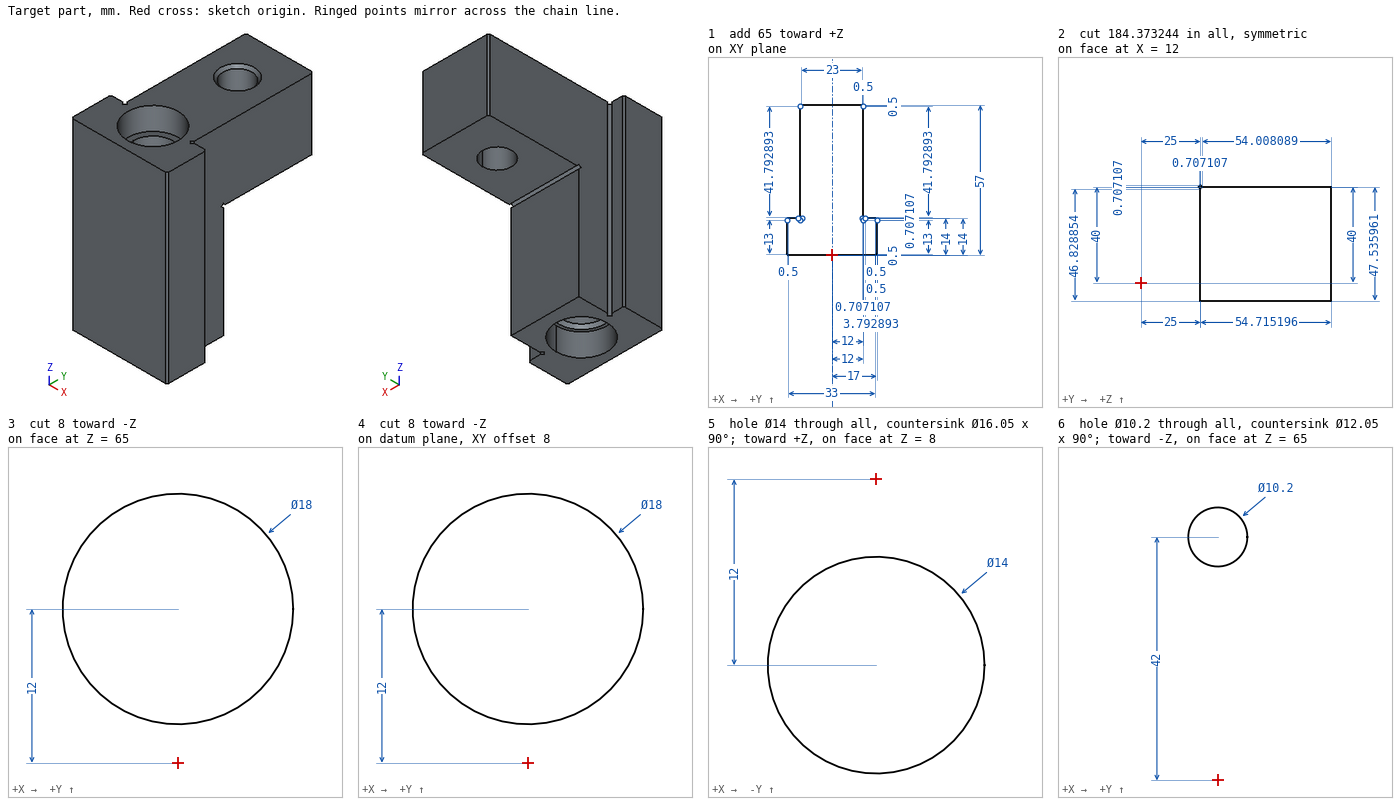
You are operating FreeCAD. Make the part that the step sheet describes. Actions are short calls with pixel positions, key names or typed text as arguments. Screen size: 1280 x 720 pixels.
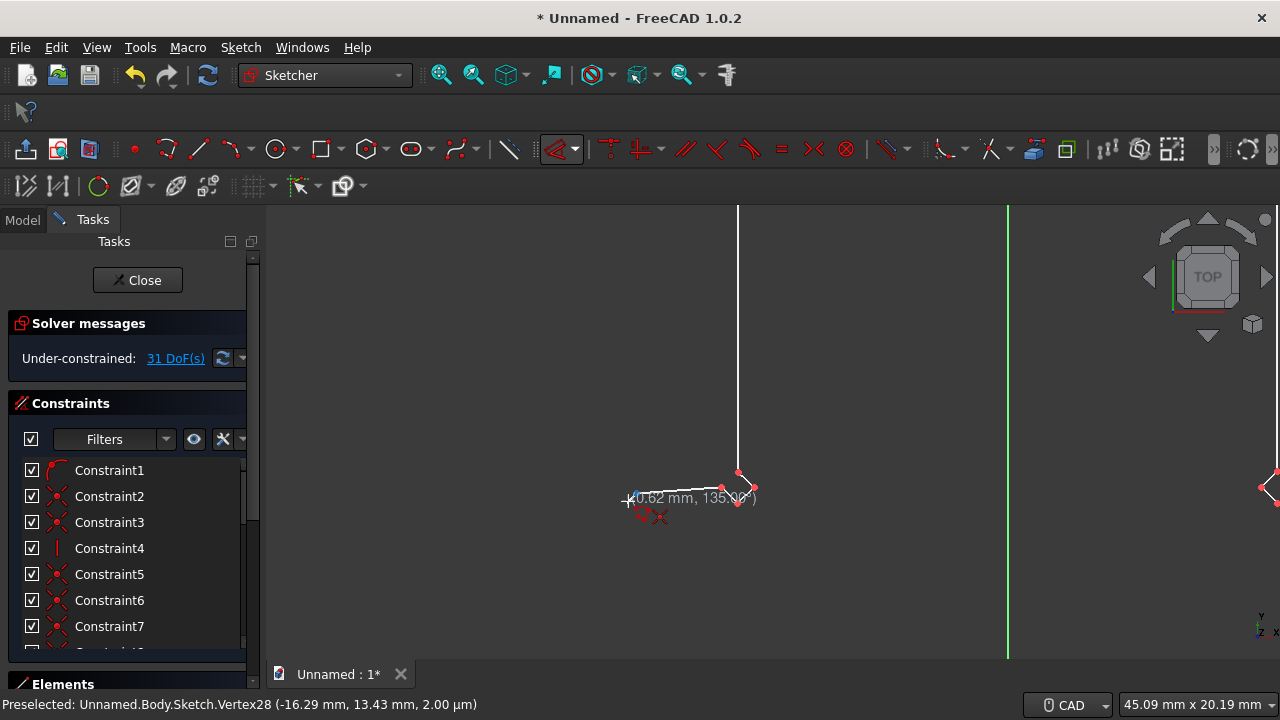
click(625, 497)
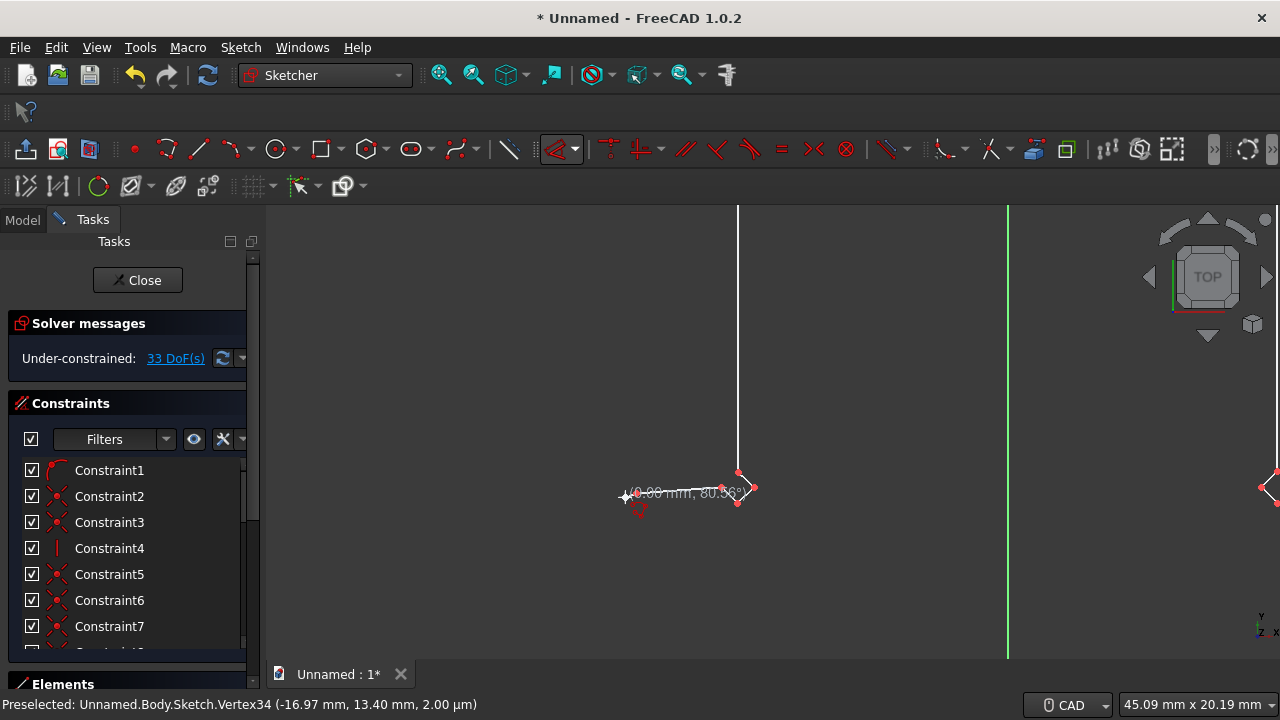
scroll(628, 501, down, 8)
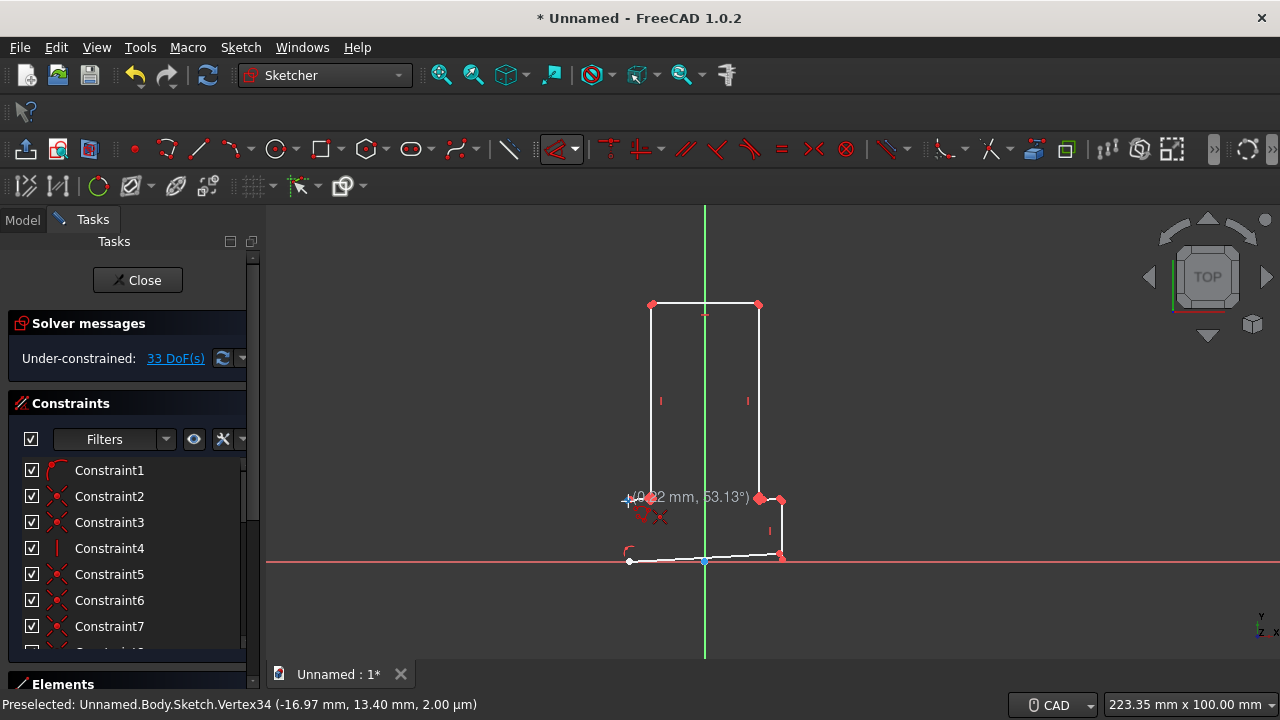
scroll(628, 560, up, 10)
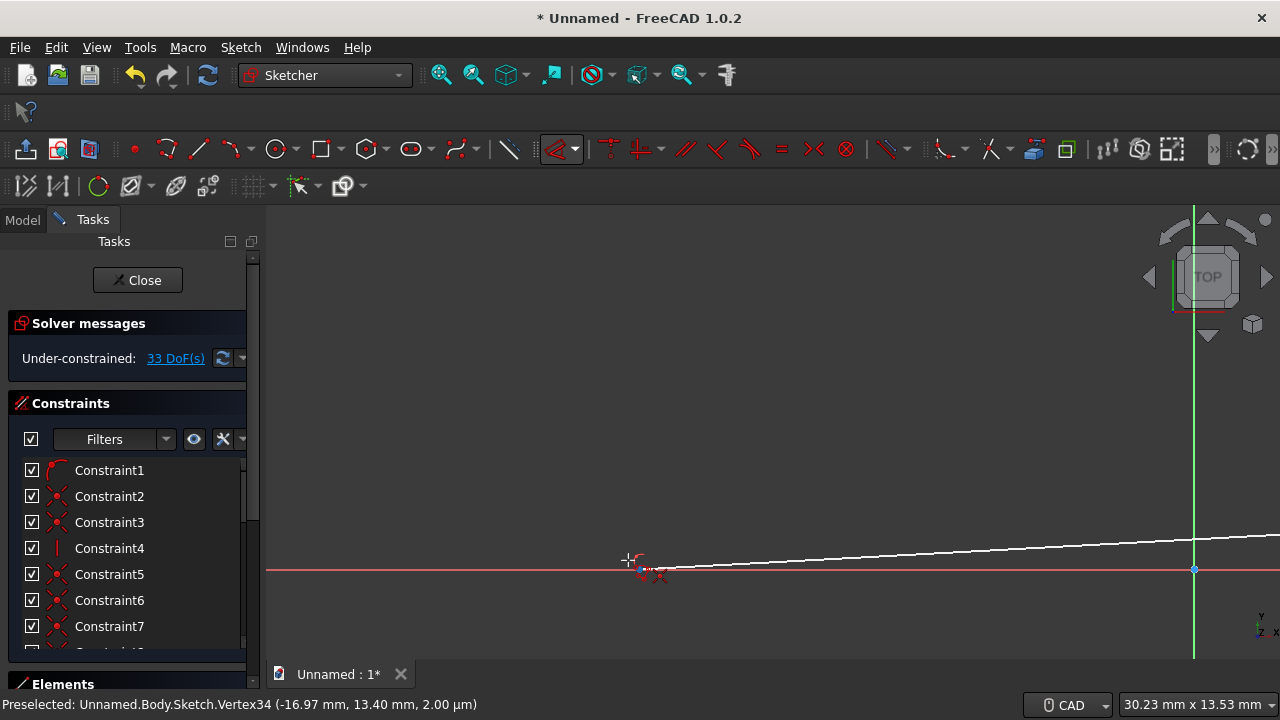
click(623, 553)
click(640, 570)
key(Escape)
key(Escape)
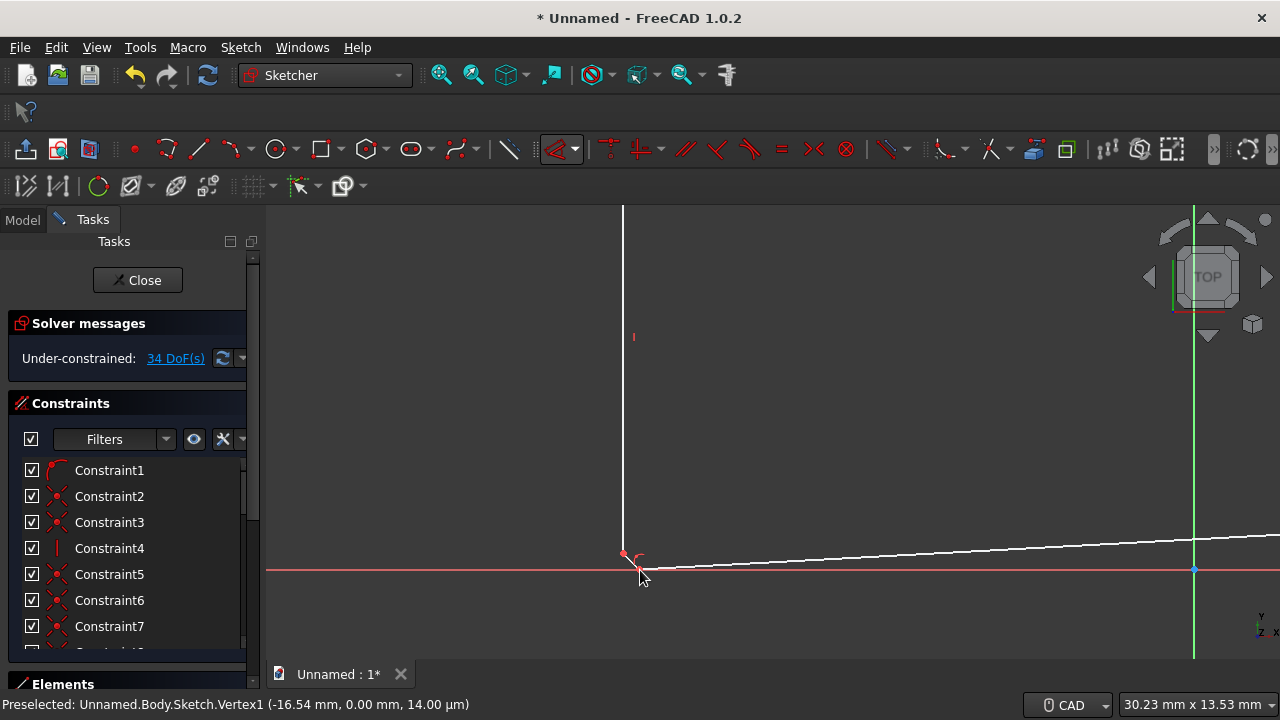
click(972, 551)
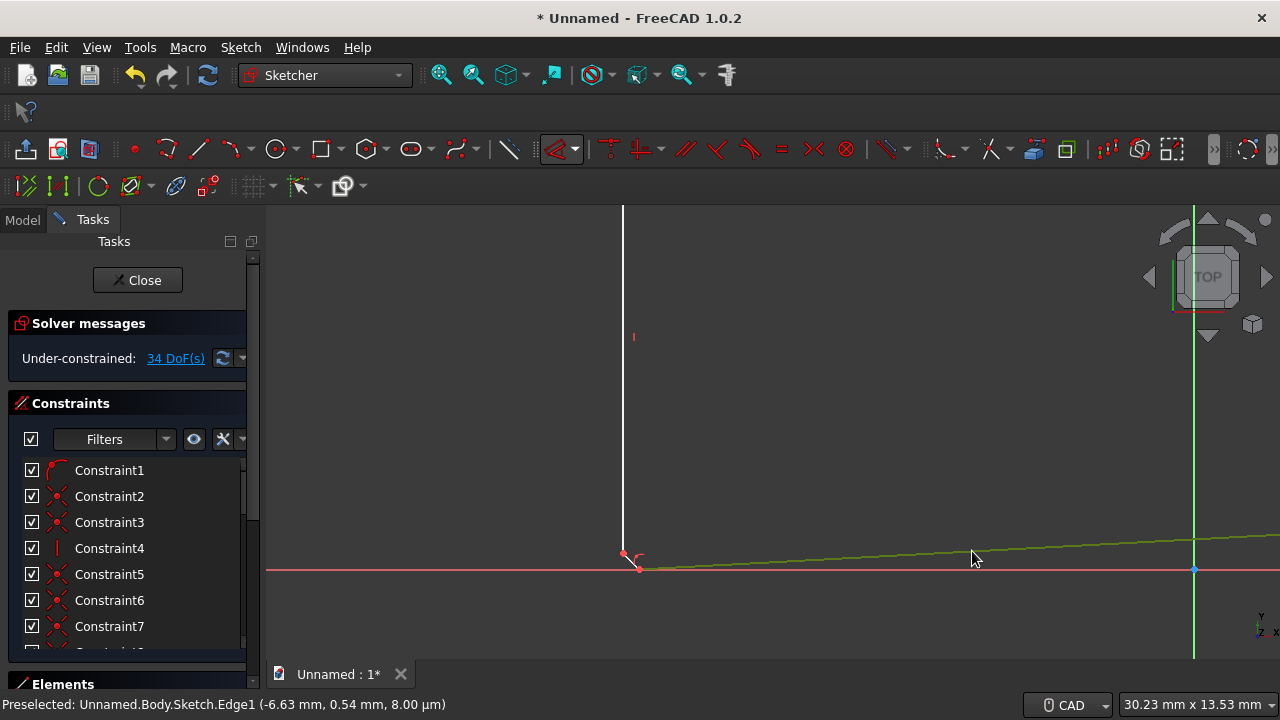
key(h)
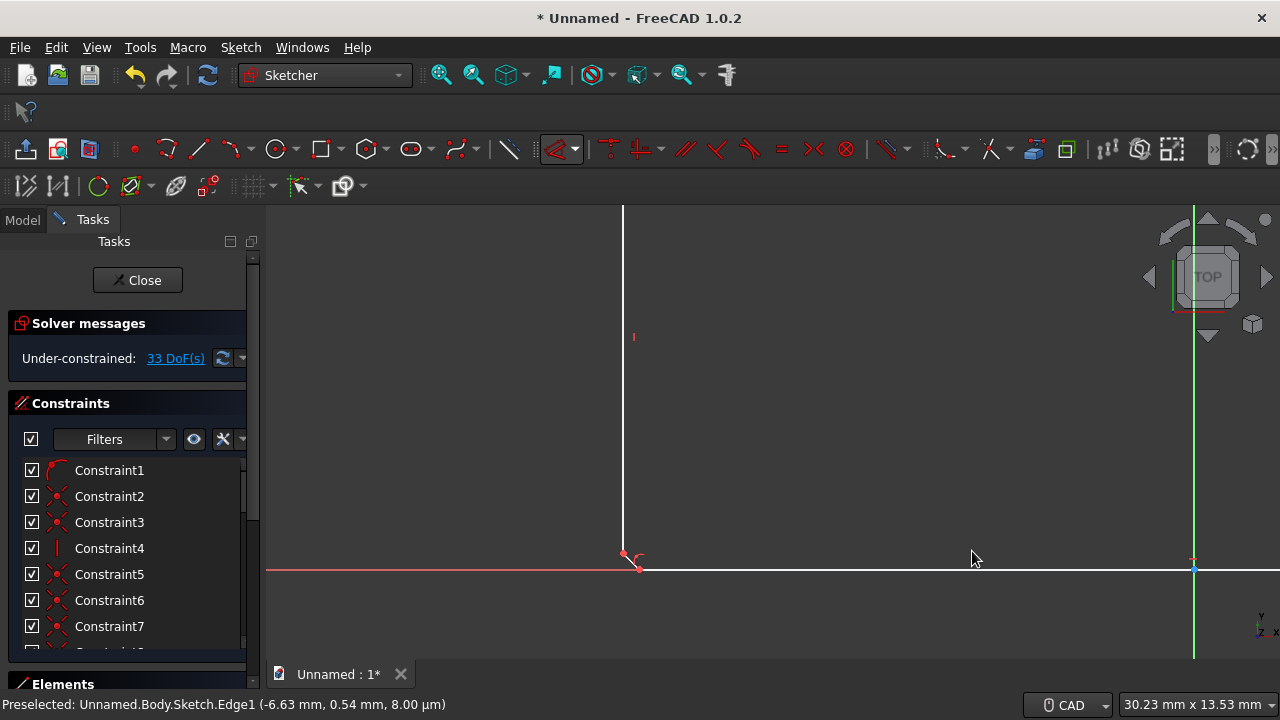
scroll(628, 560, down, 10)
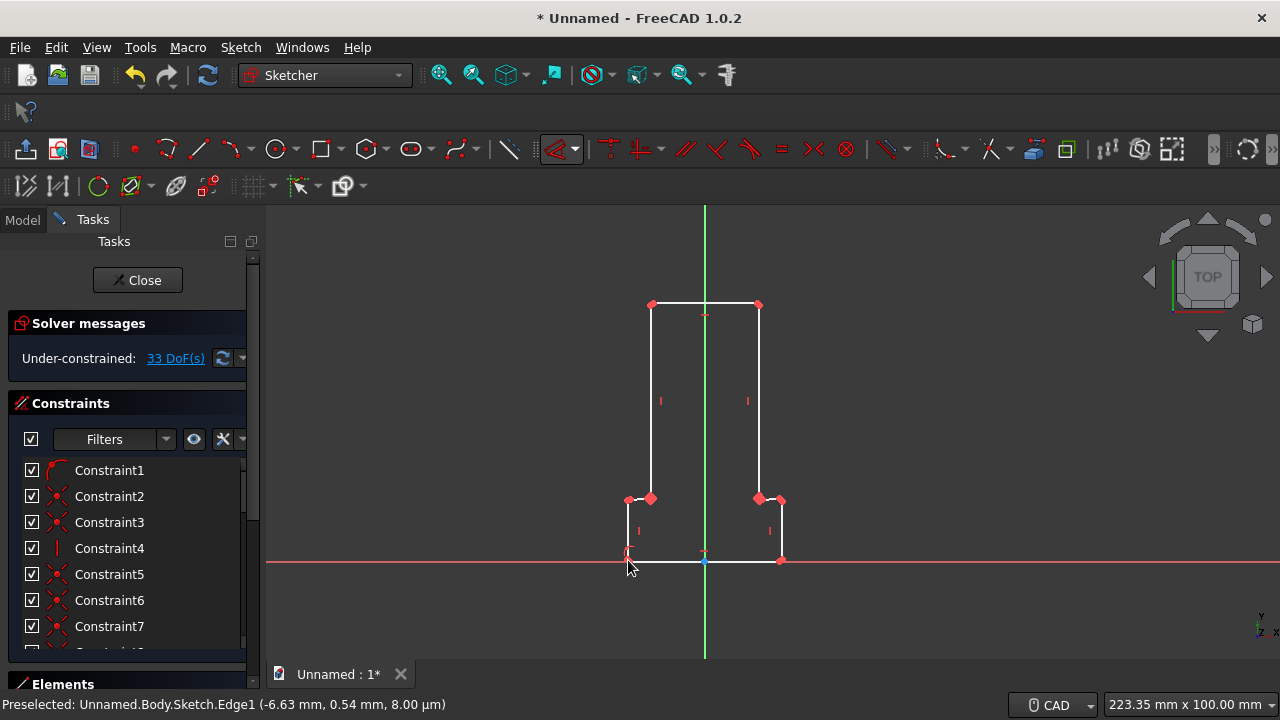
scroll(775, 499, up, 6)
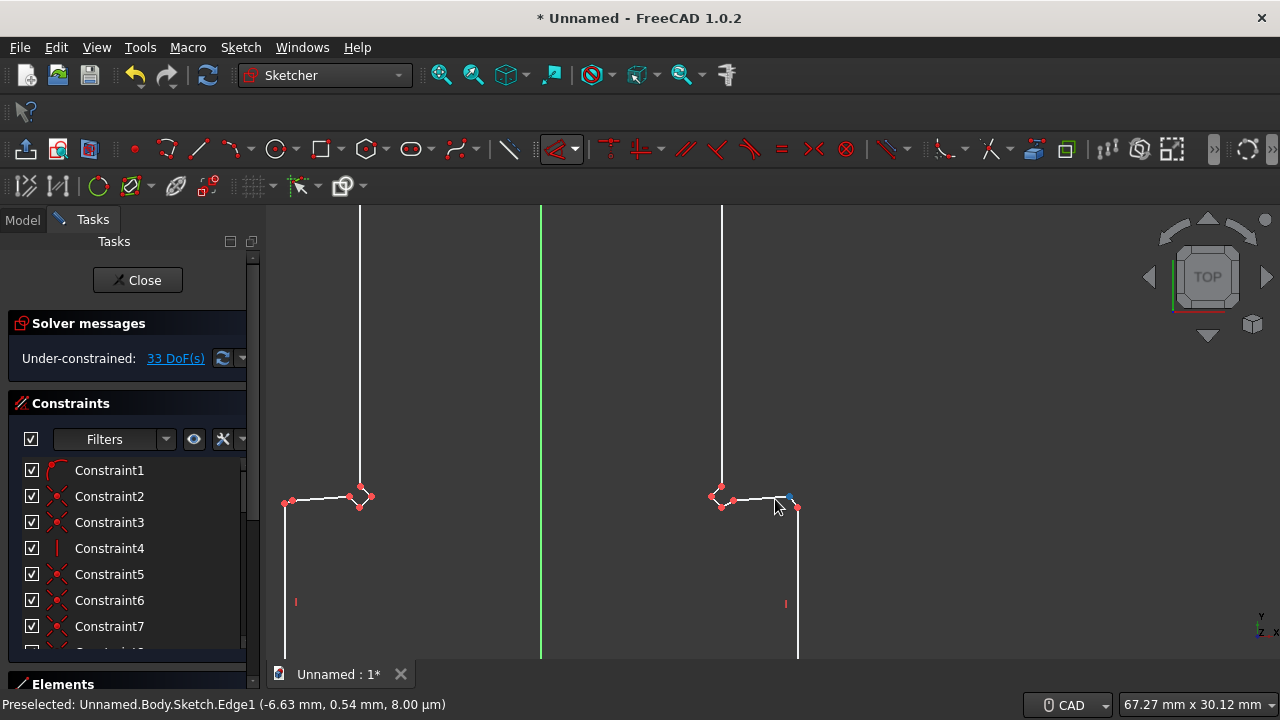
click(773, 498)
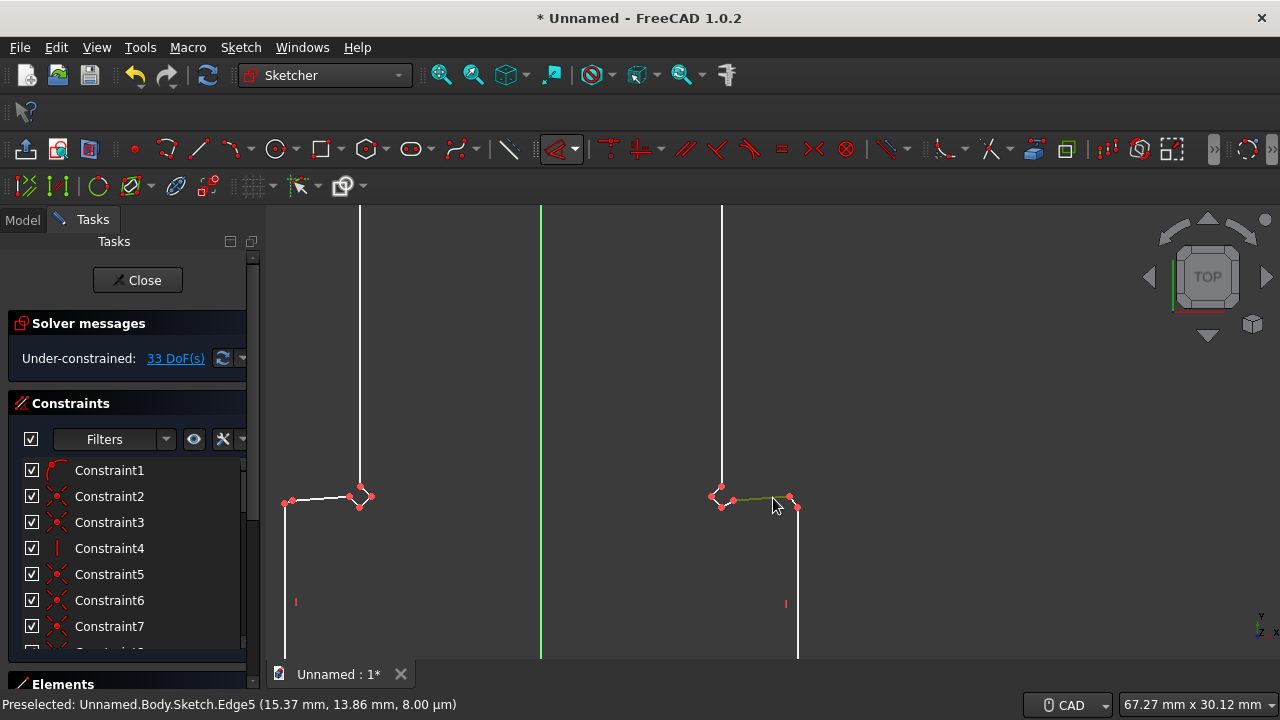
key(h)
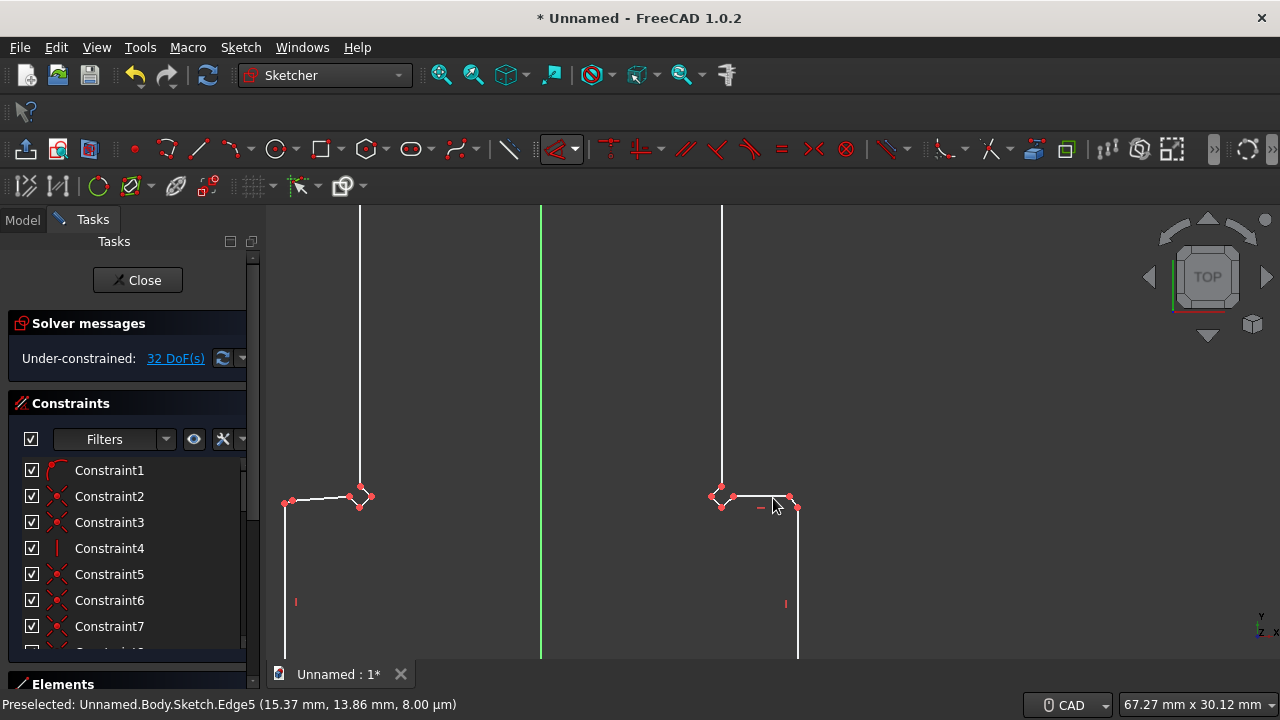
click(332, 498)